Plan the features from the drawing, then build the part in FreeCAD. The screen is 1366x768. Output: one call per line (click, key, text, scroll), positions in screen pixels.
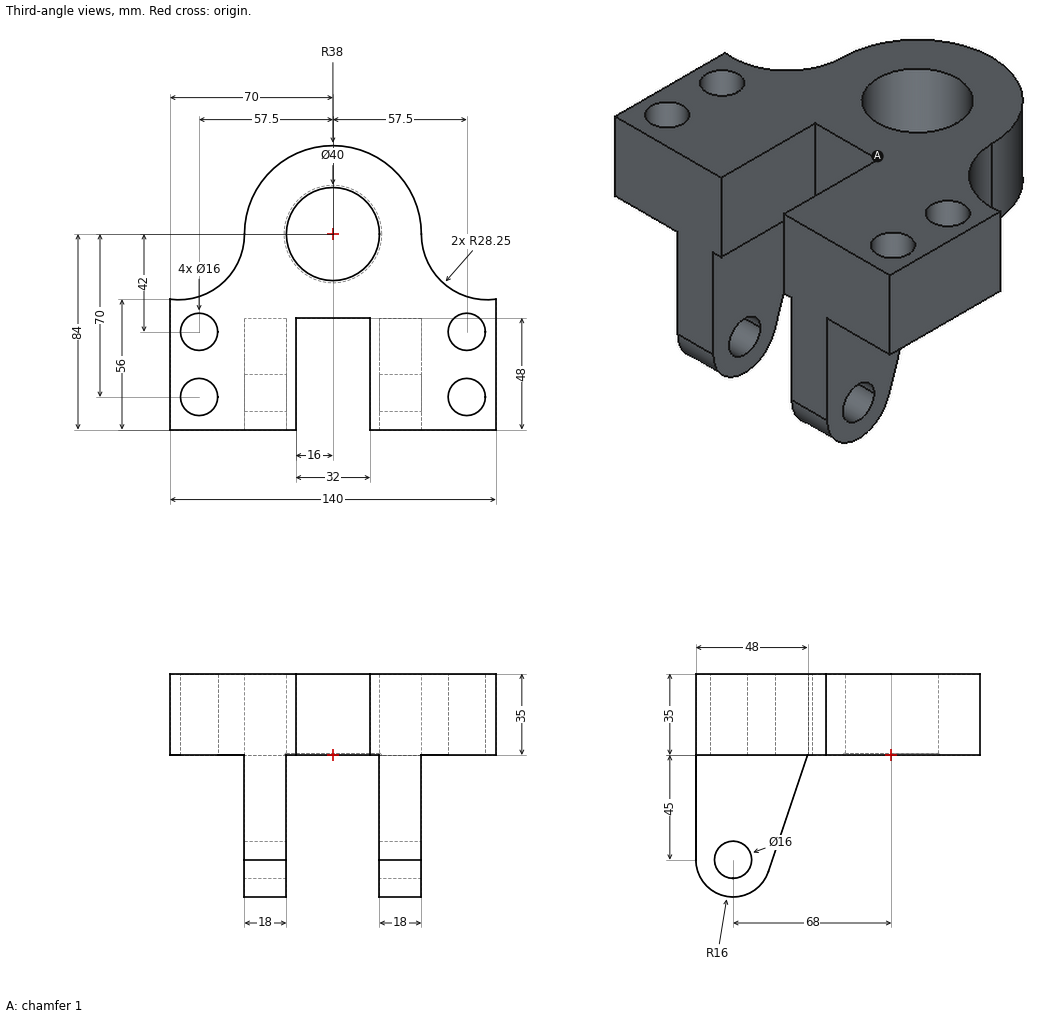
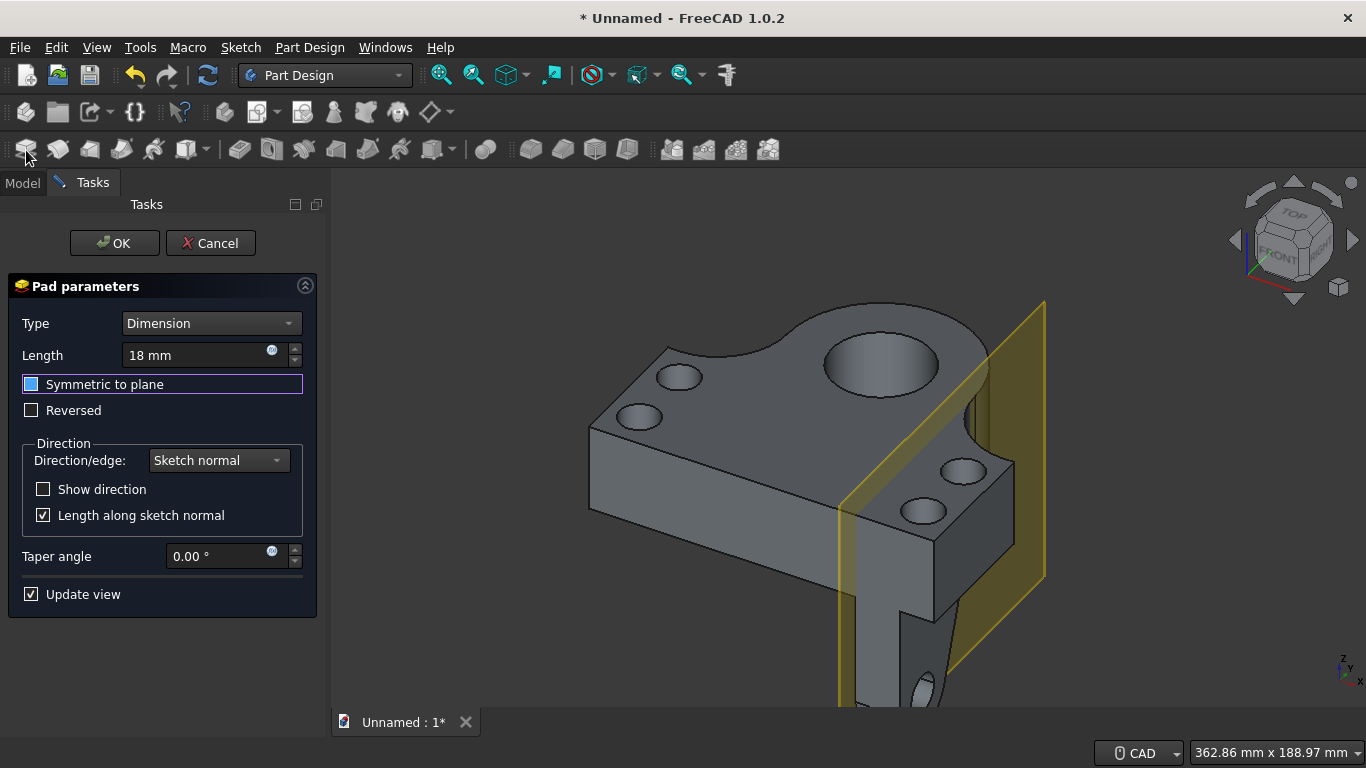
click(30, 410)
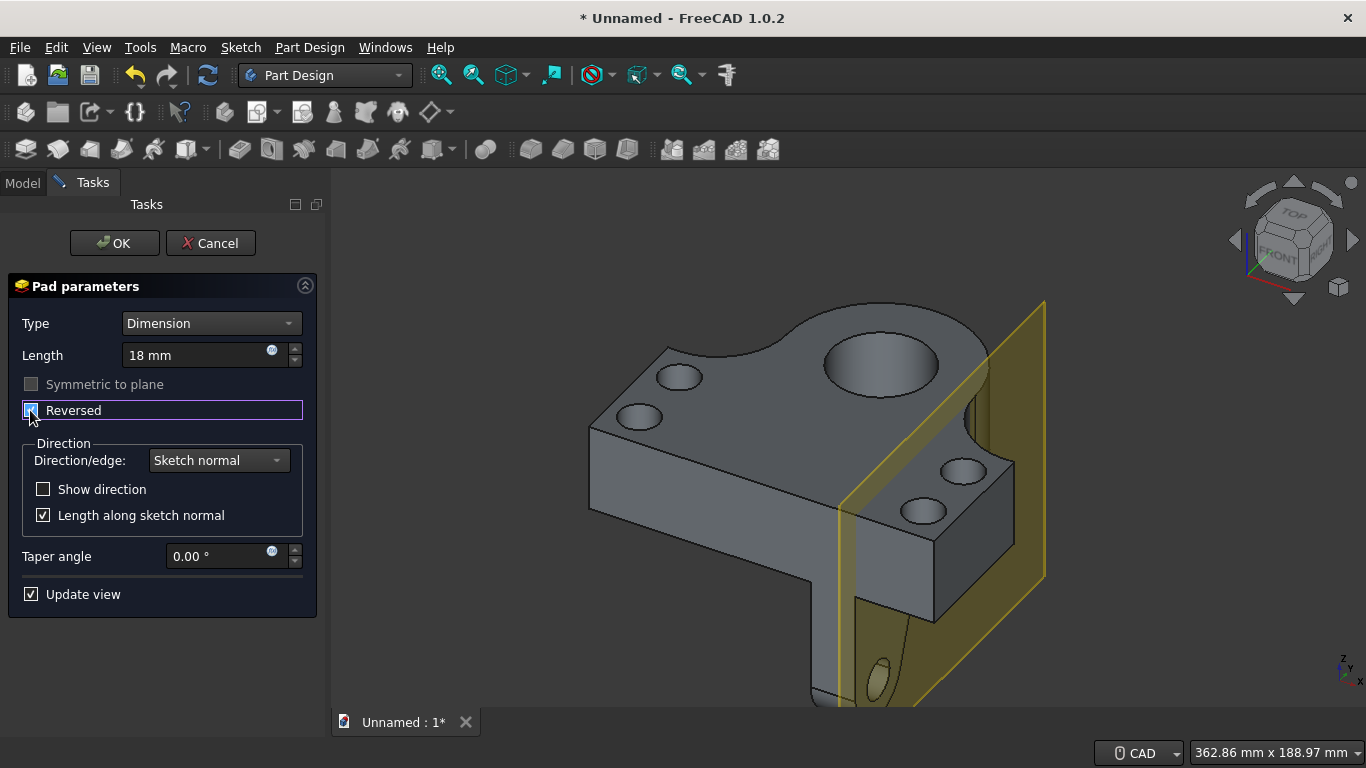
click(115, 243)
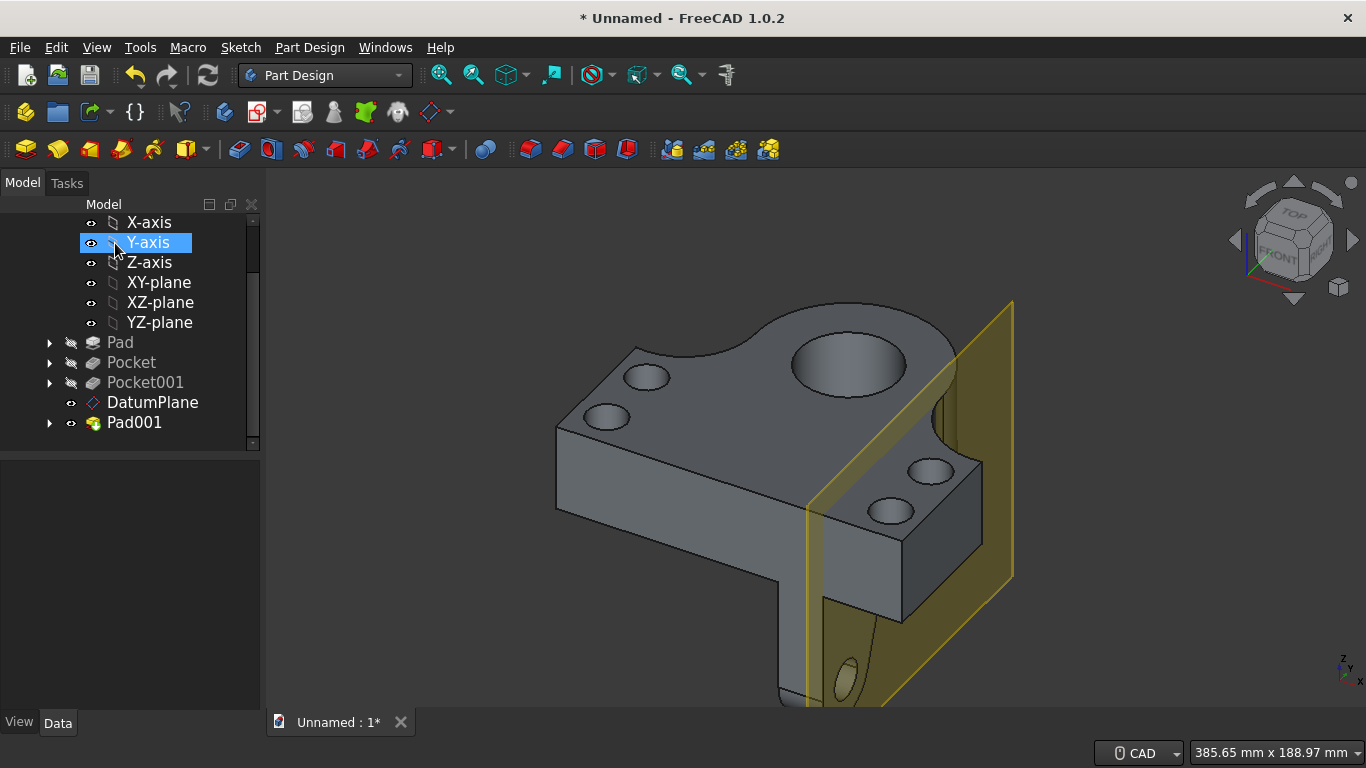
click(116, 403)
key(space)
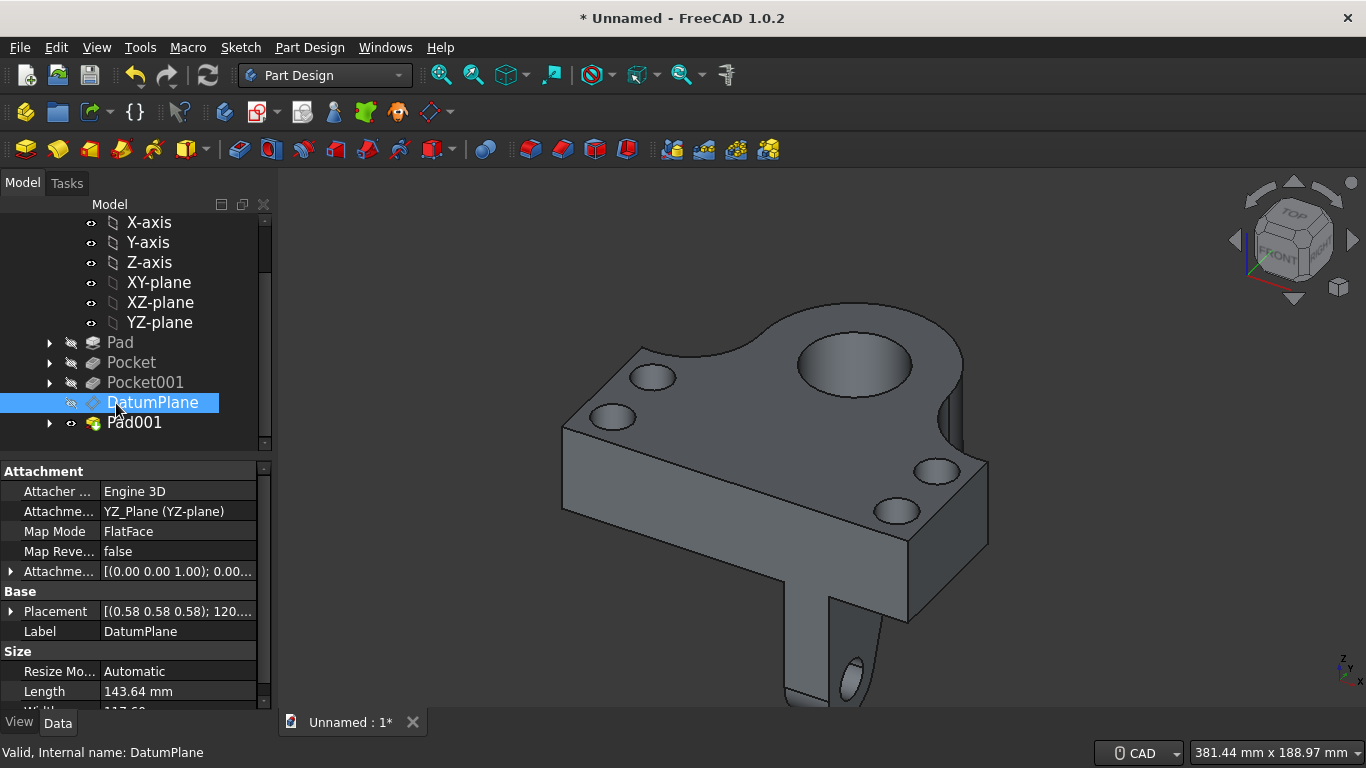
click(442, 76)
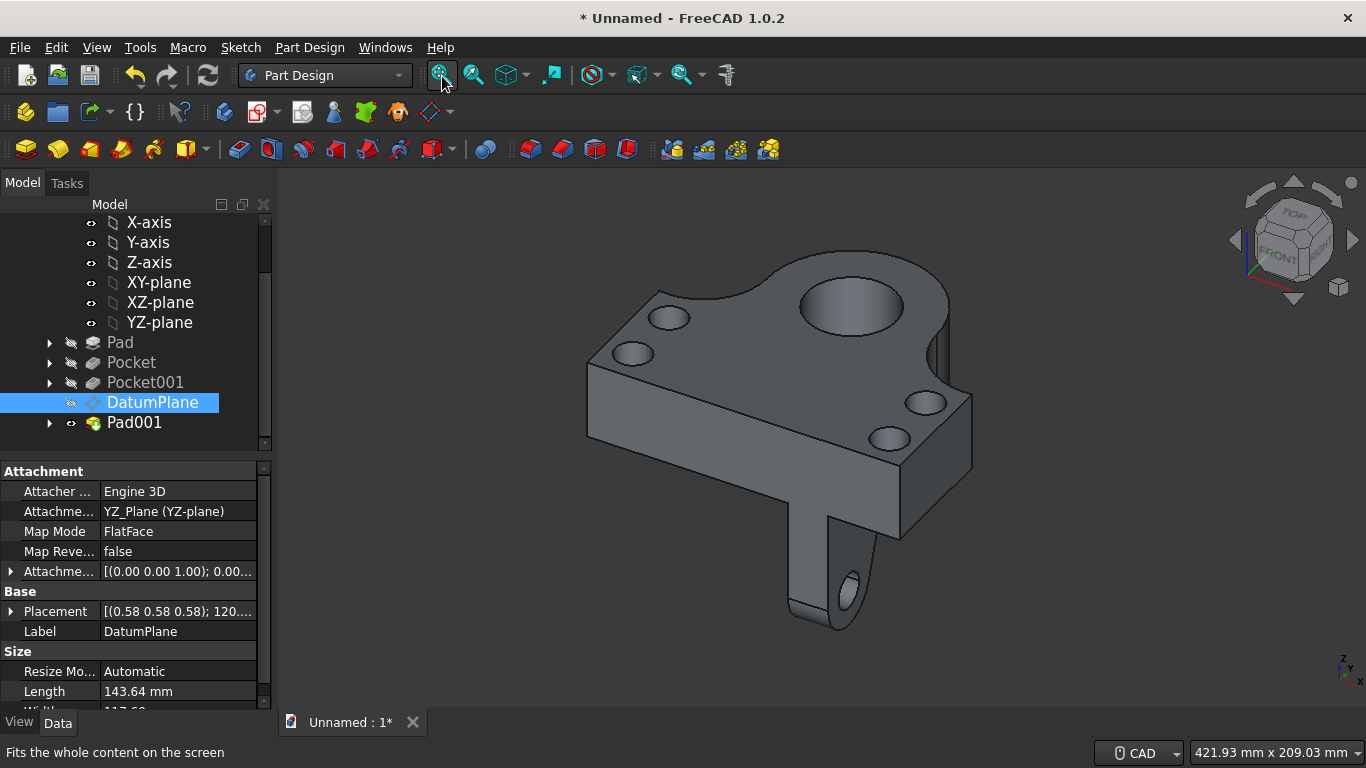
scroll(160, 318, down, 3)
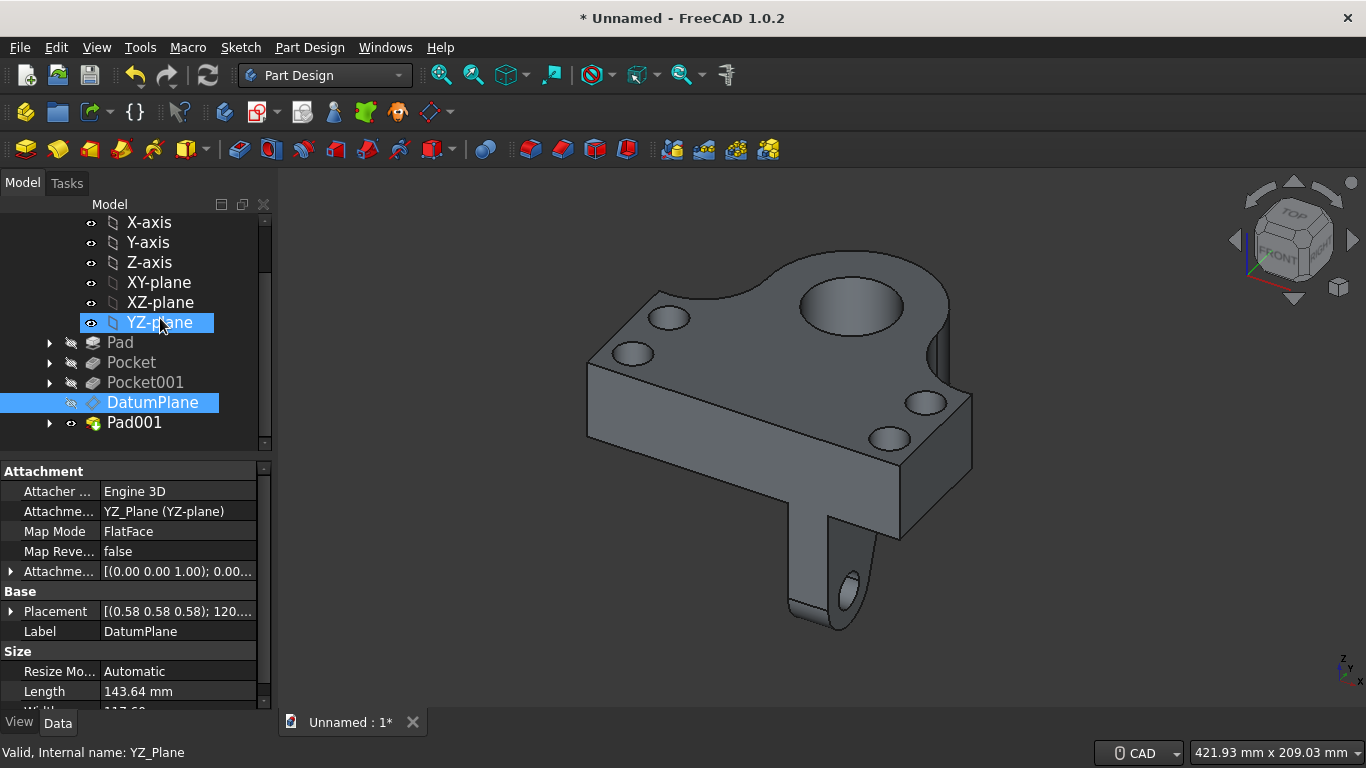
scroll(160, 318, up, 15)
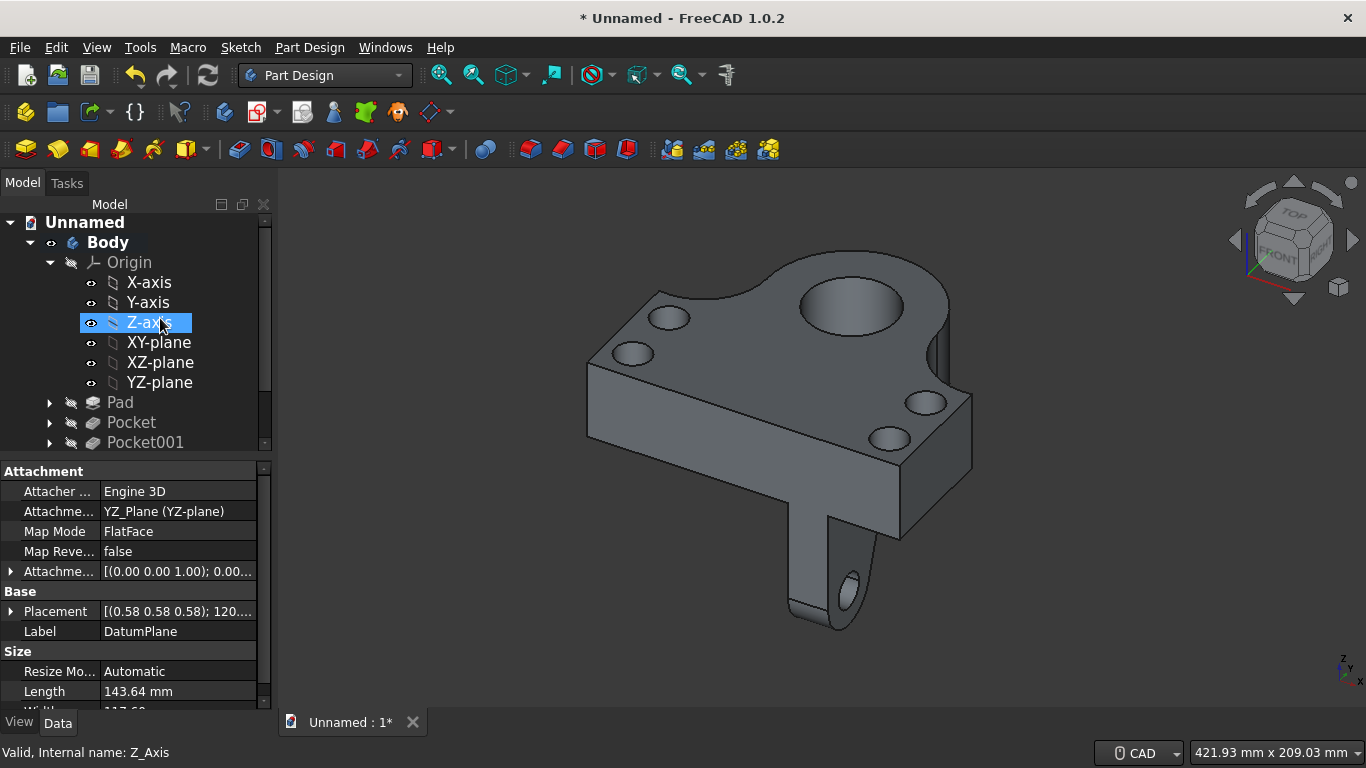
click(136, 383)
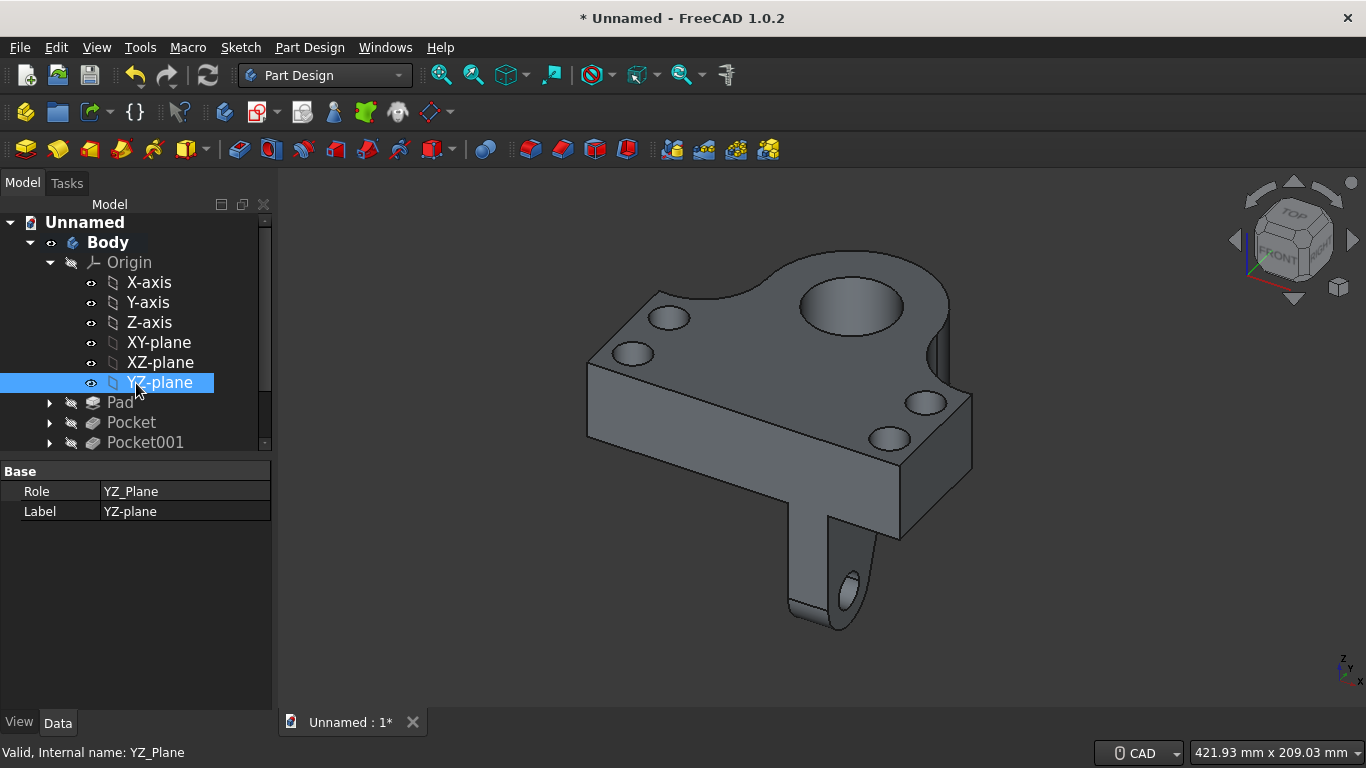
click(430, 112)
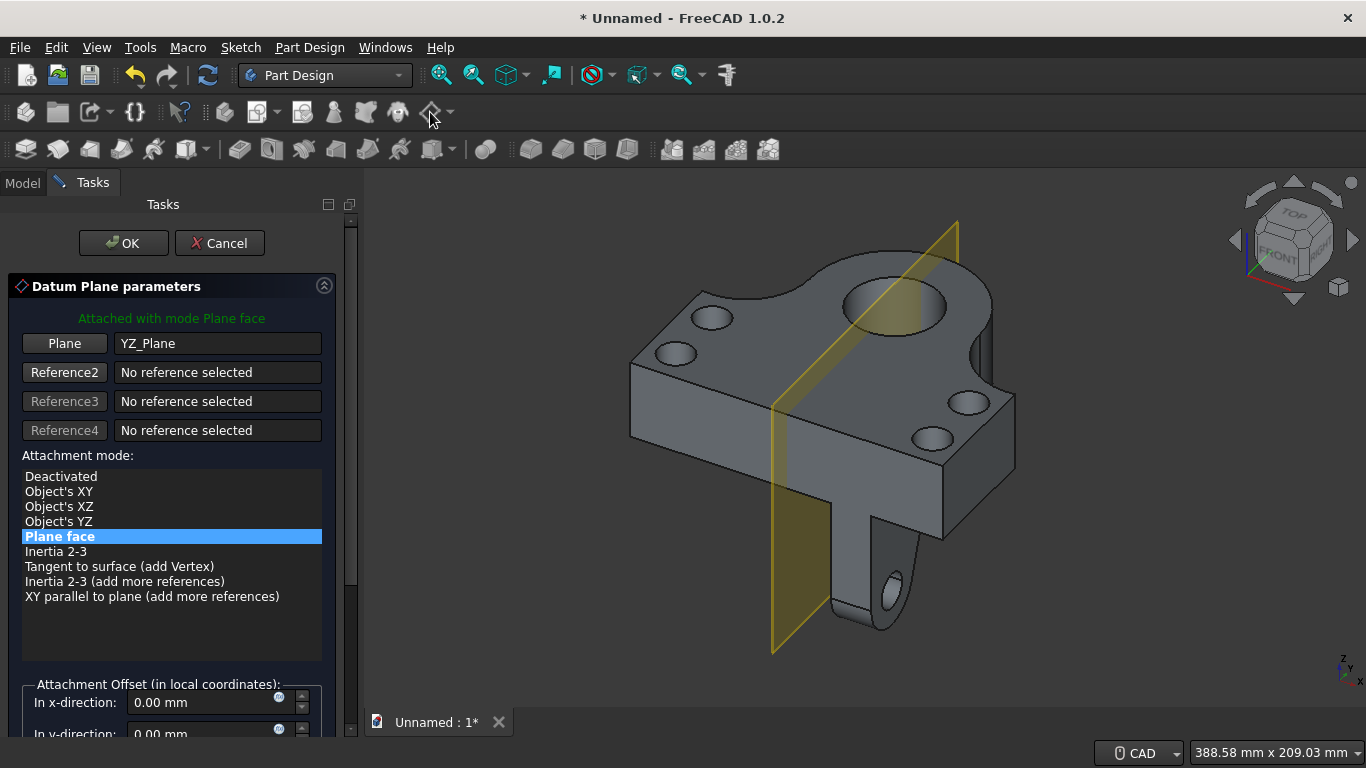
scroll(351, 475, down, 2)